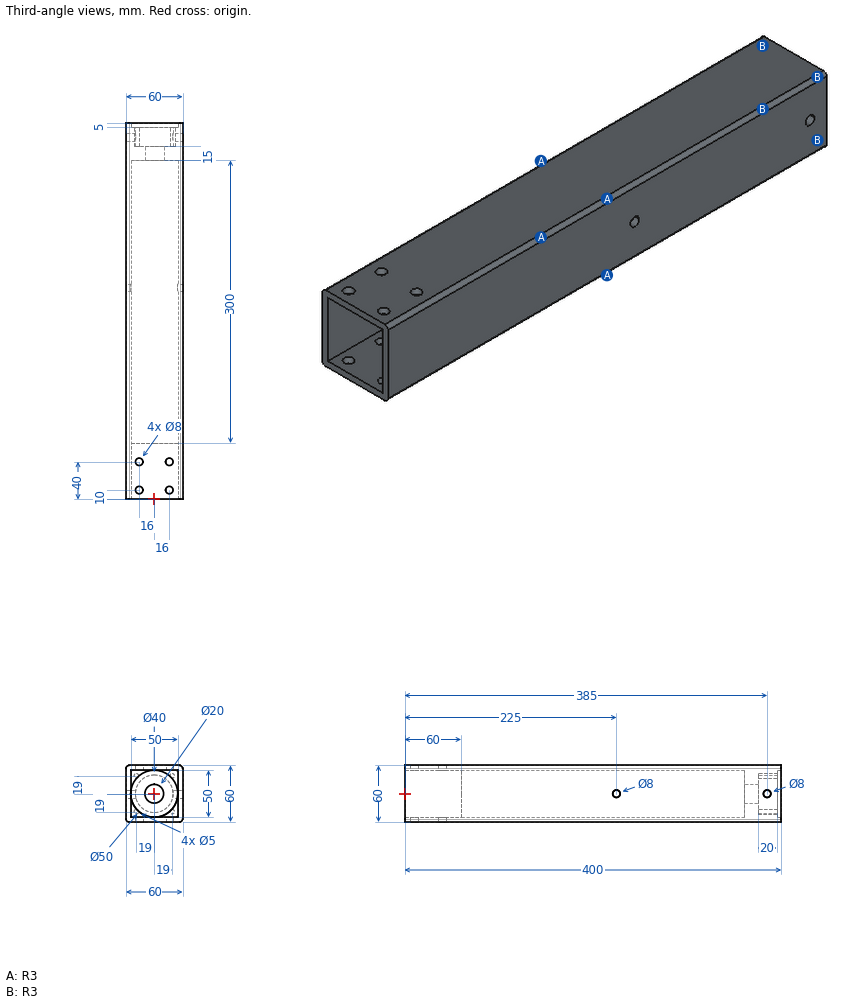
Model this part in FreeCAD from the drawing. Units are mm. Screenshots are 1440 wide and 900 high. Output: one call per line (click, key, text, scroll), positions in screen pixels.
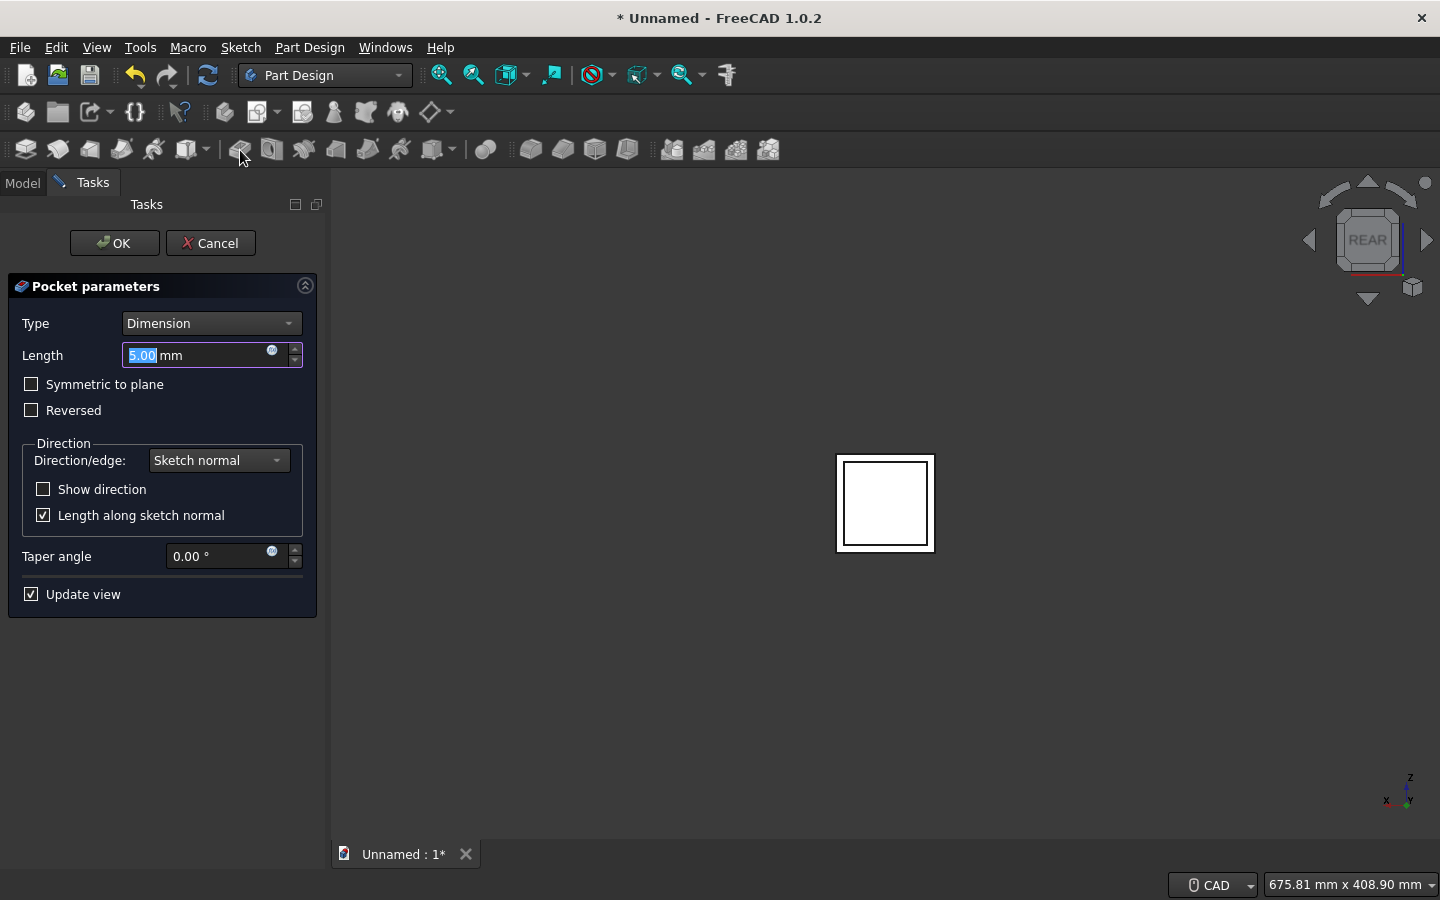
text(5)
key(Tab)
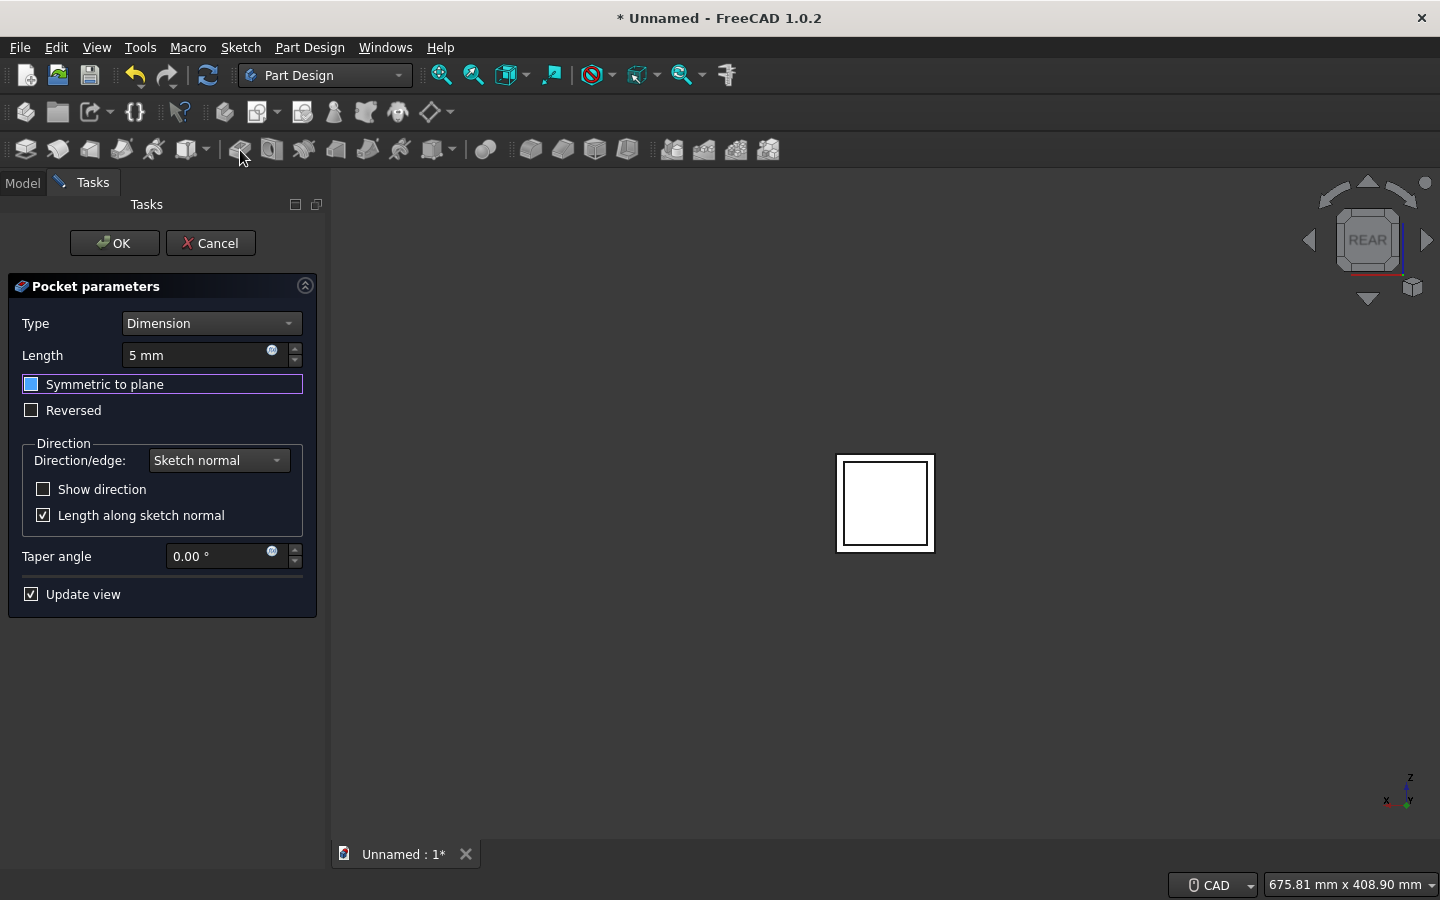
click(115, 243)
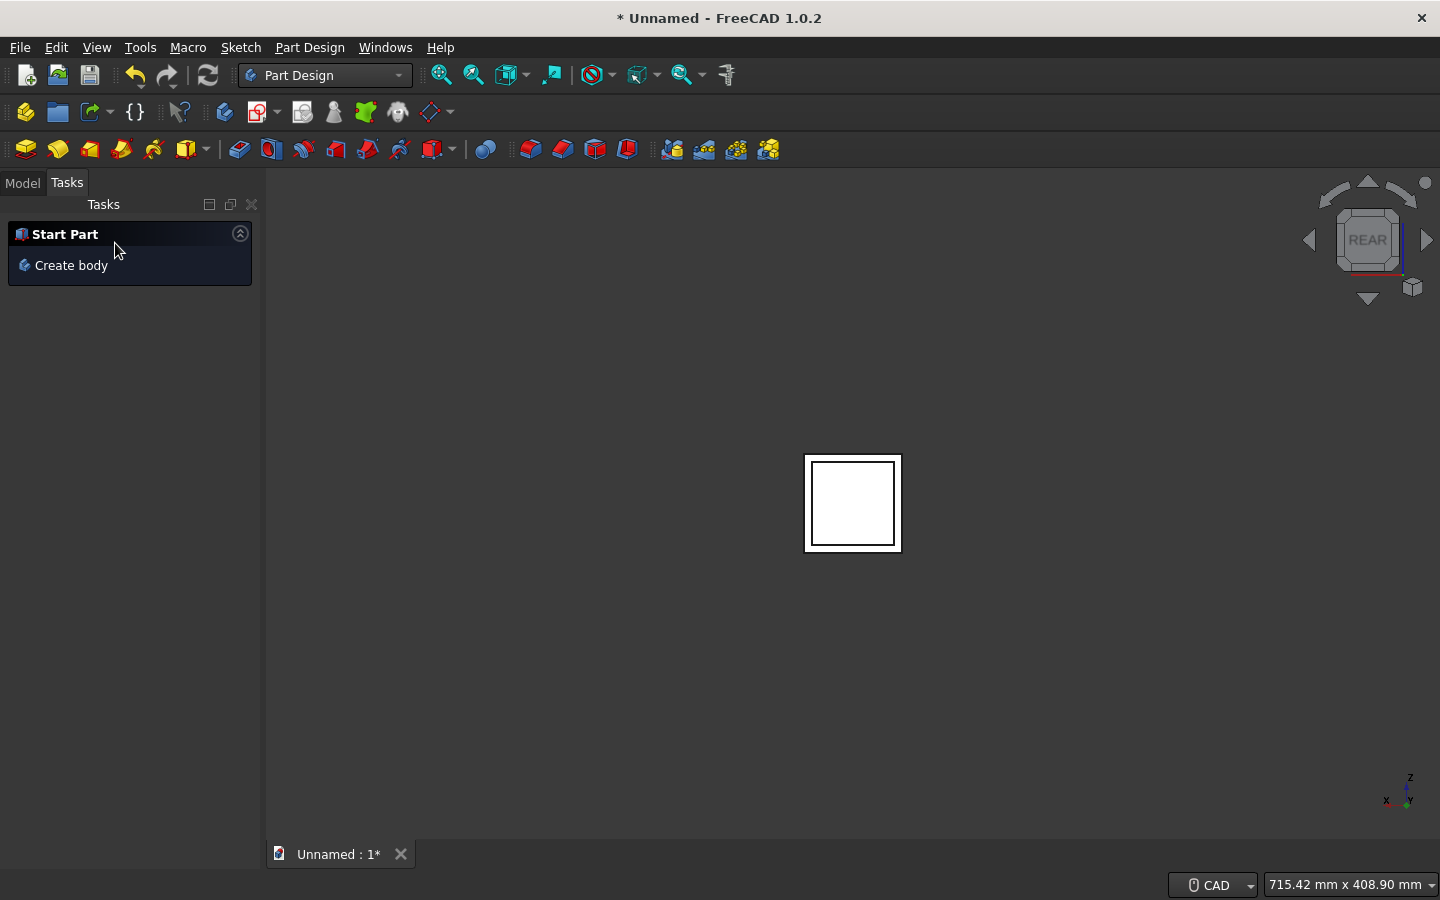
key(v)
key(f)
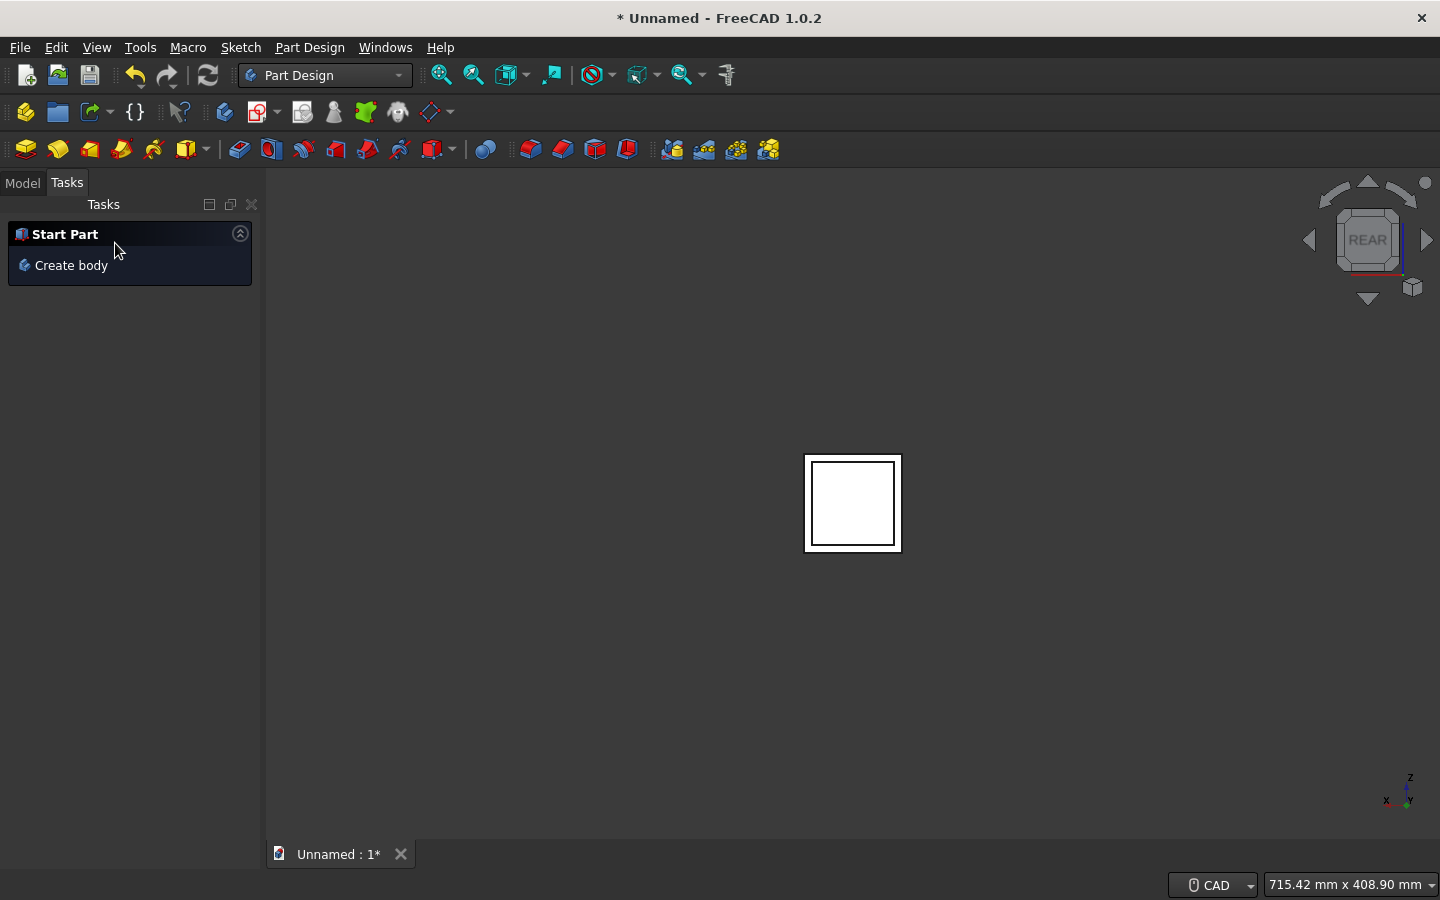
click(853, 502)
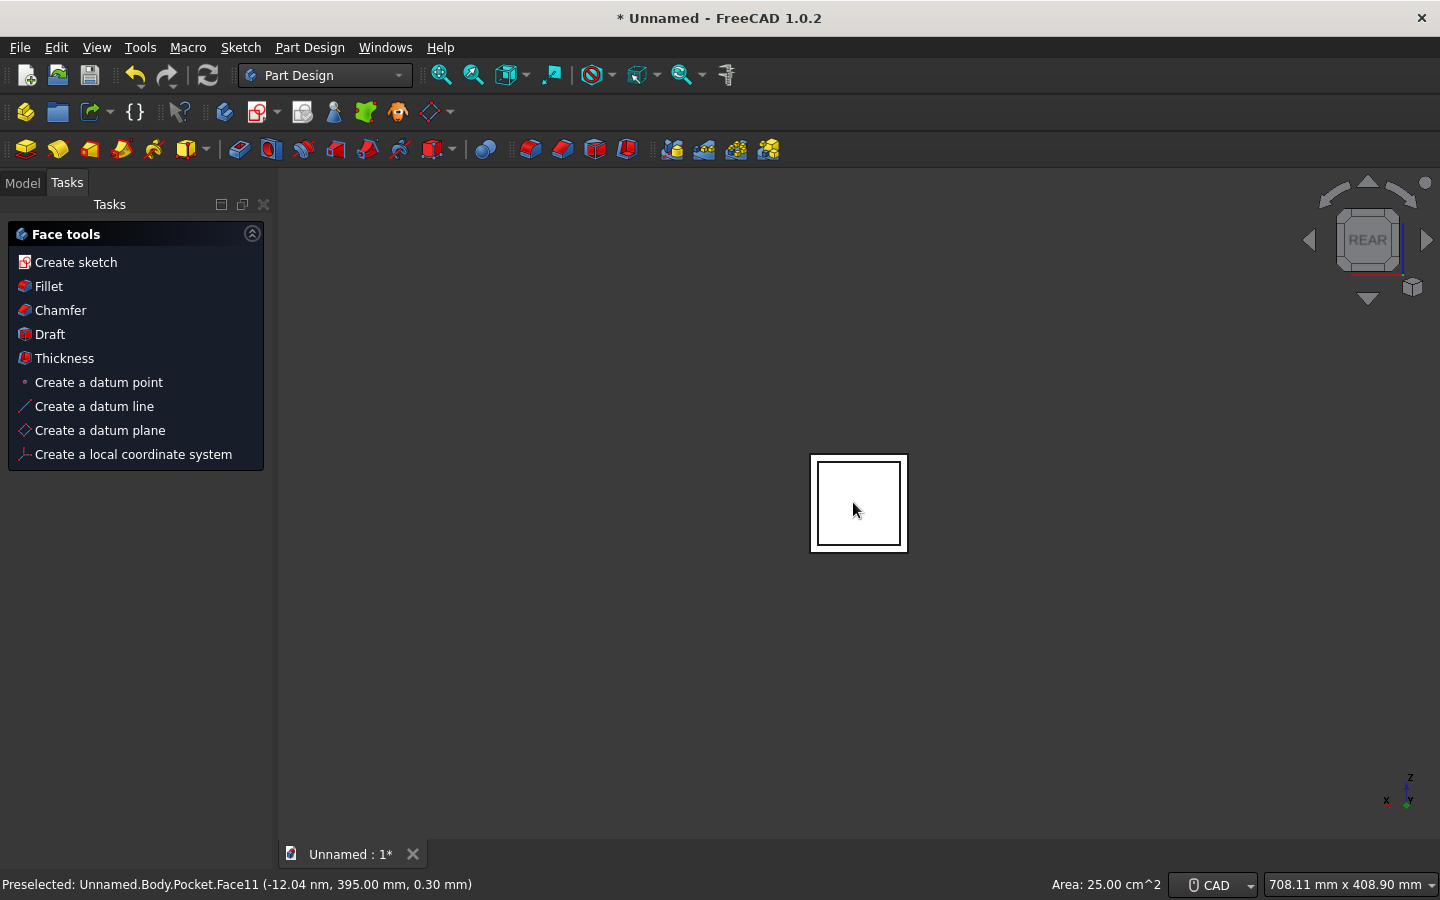
click(258, 112)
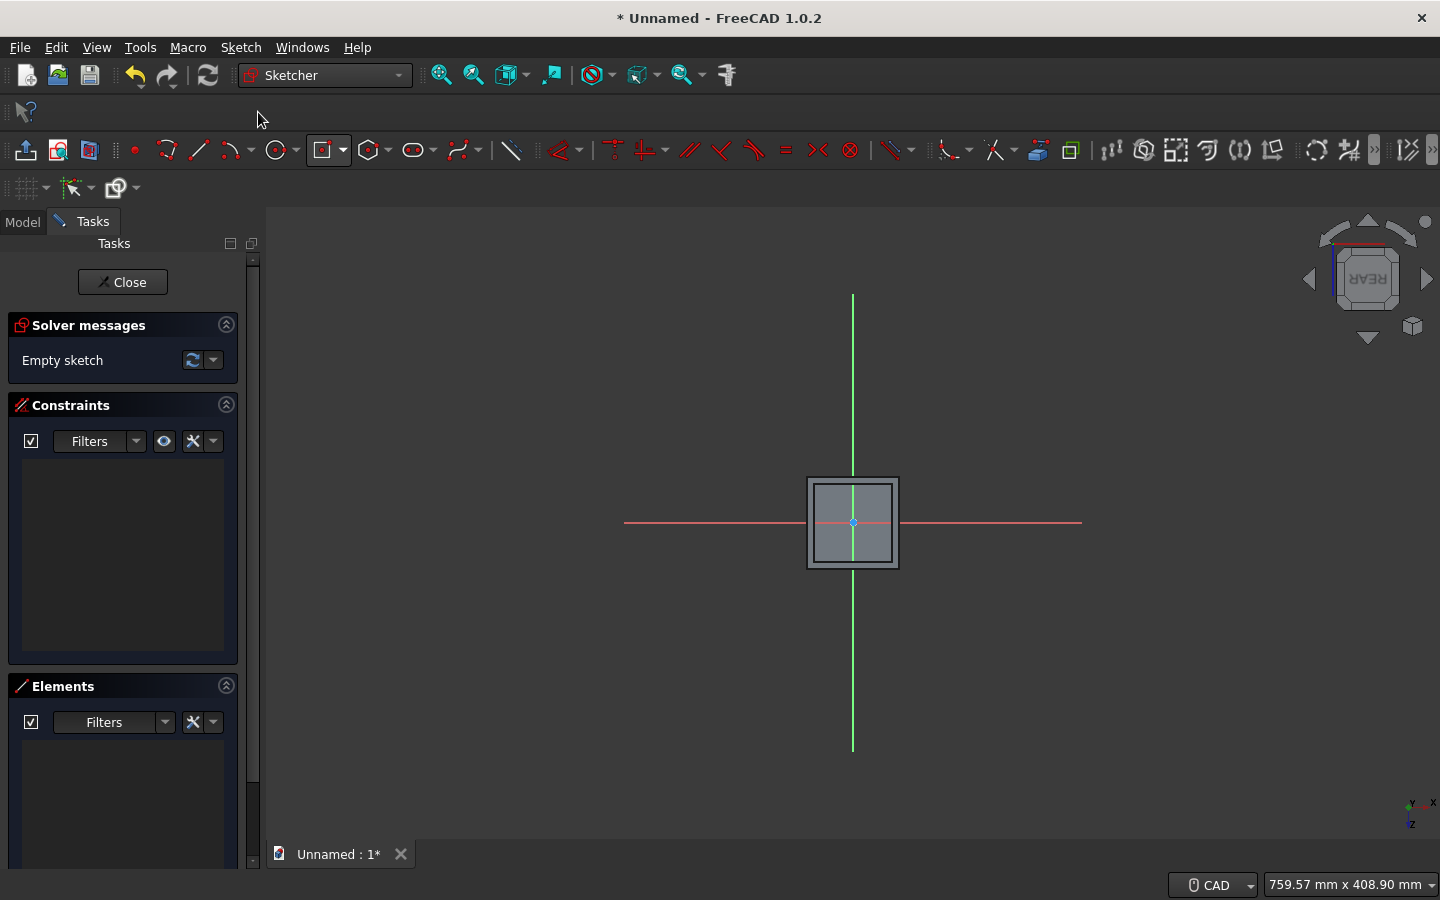
scroll(867, 523, up, 9)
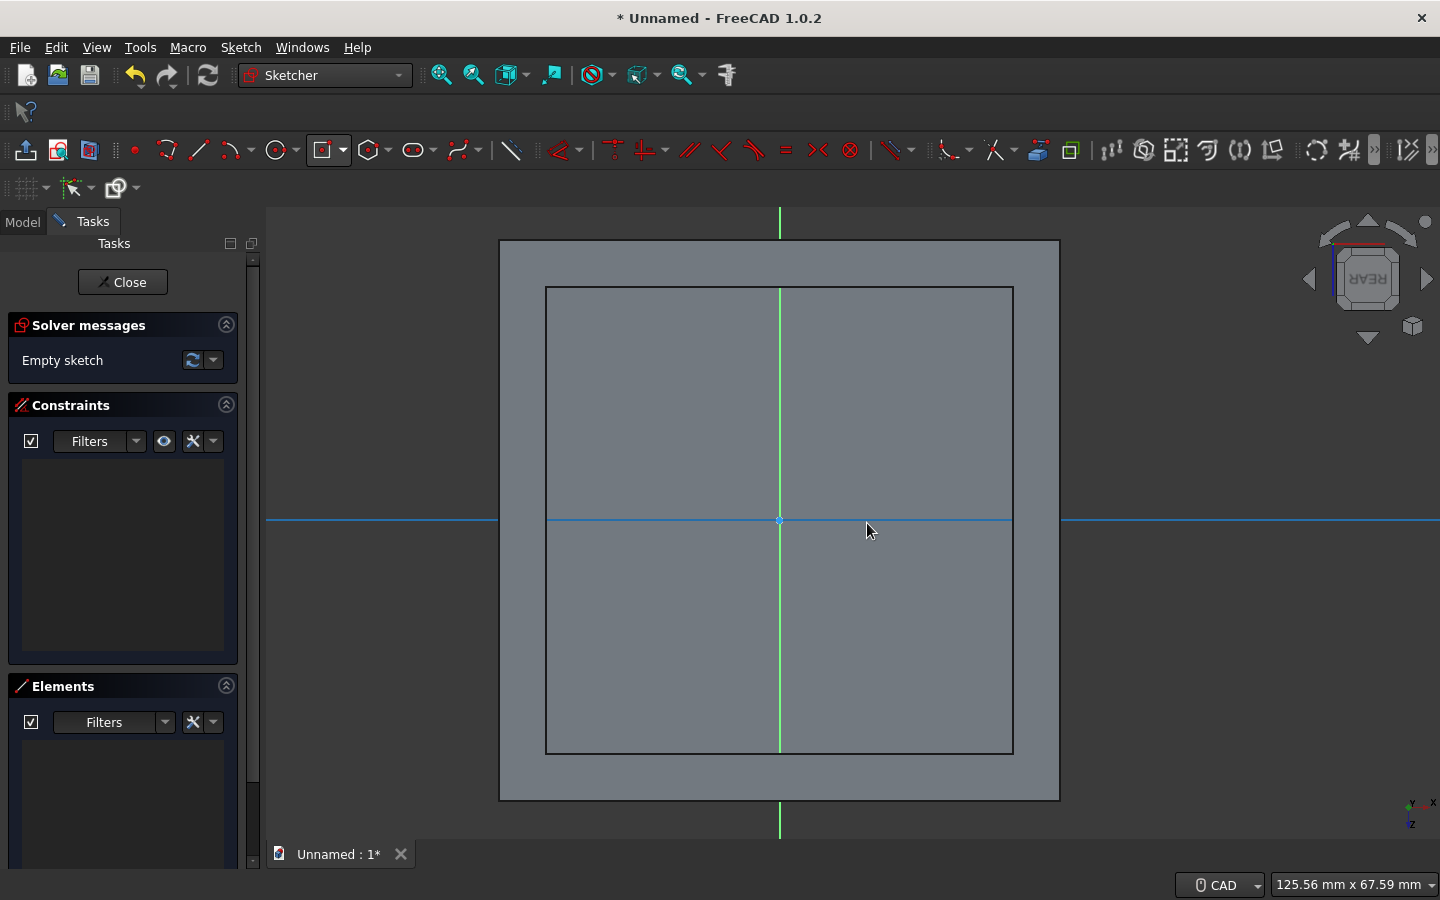
click(276, 150)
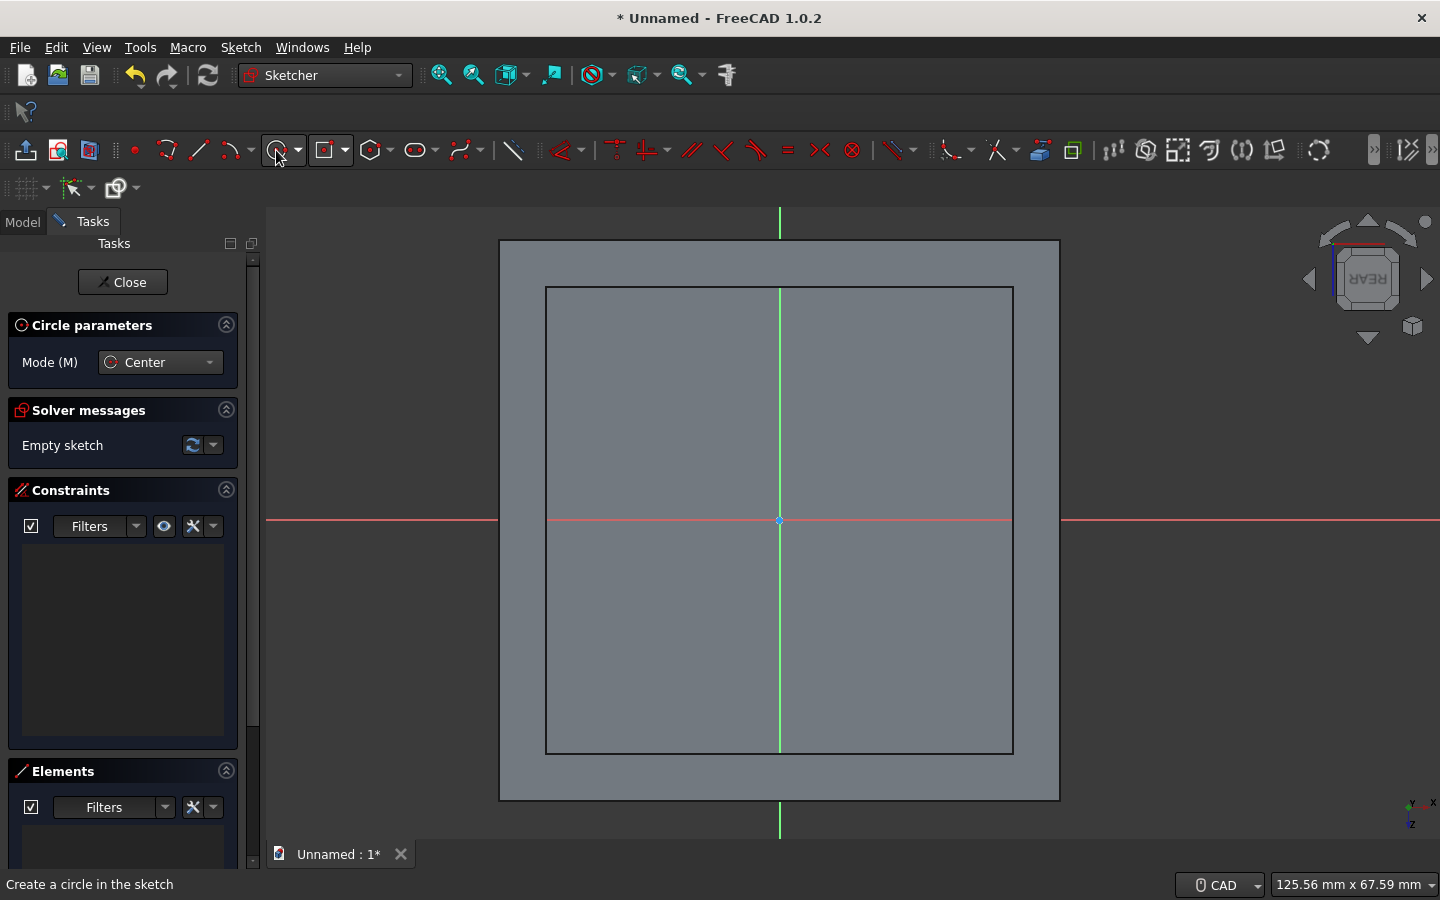
click(780, 520)
move(912, 388)